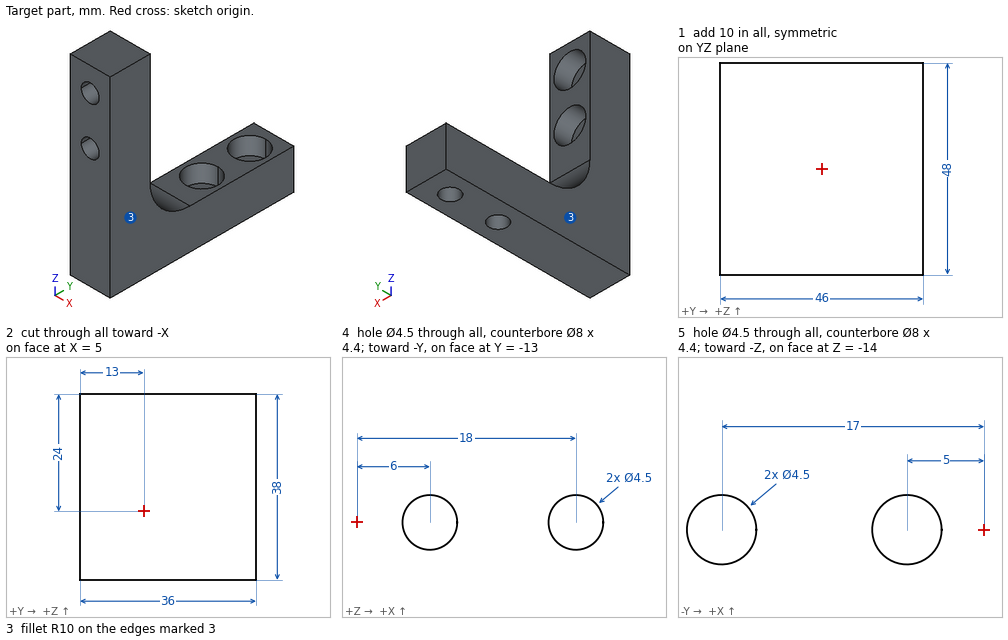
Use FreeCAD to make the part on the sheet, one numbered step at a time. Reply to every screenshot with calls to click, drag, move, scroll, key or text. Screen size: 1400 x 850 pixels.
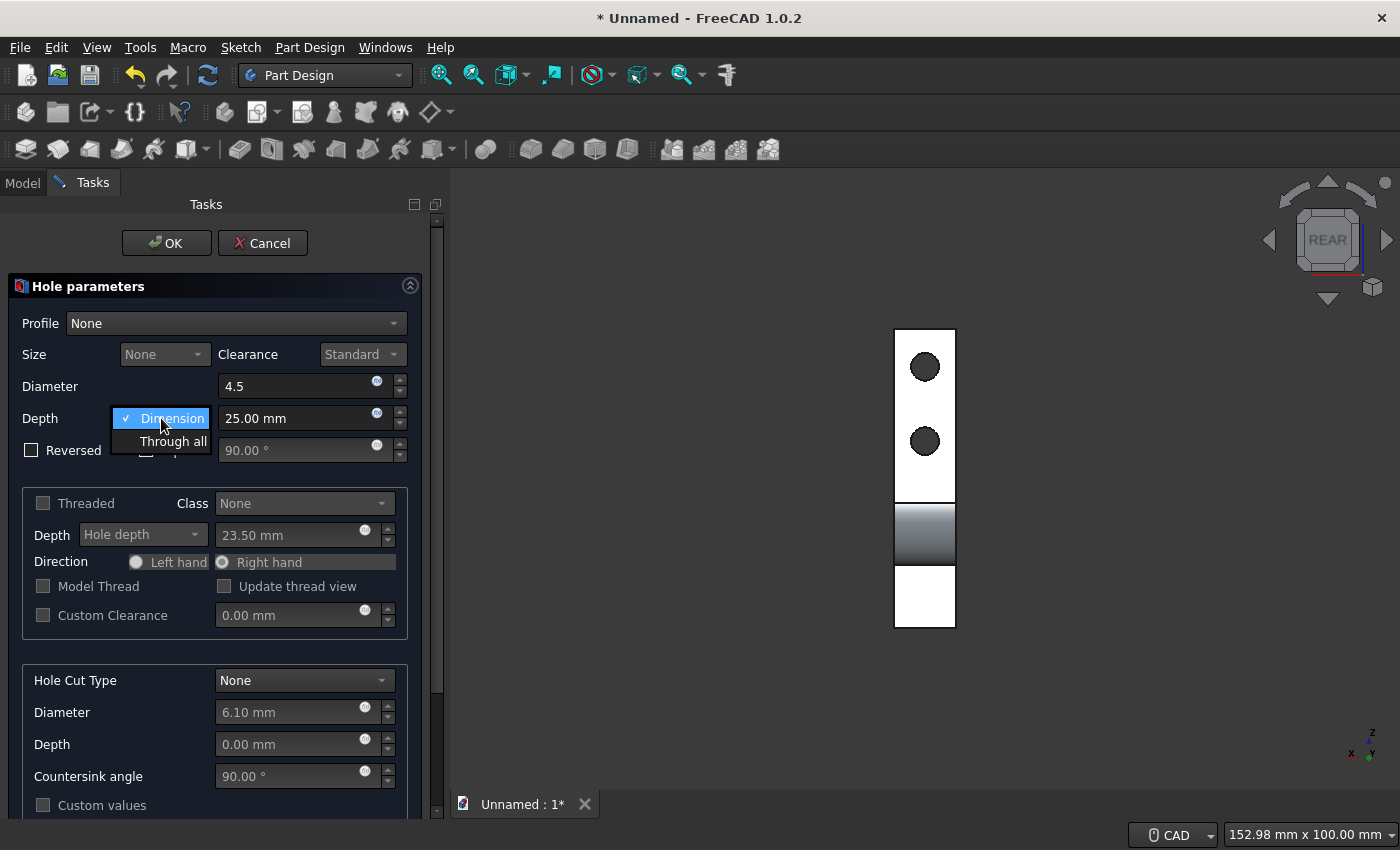
click(160, 442)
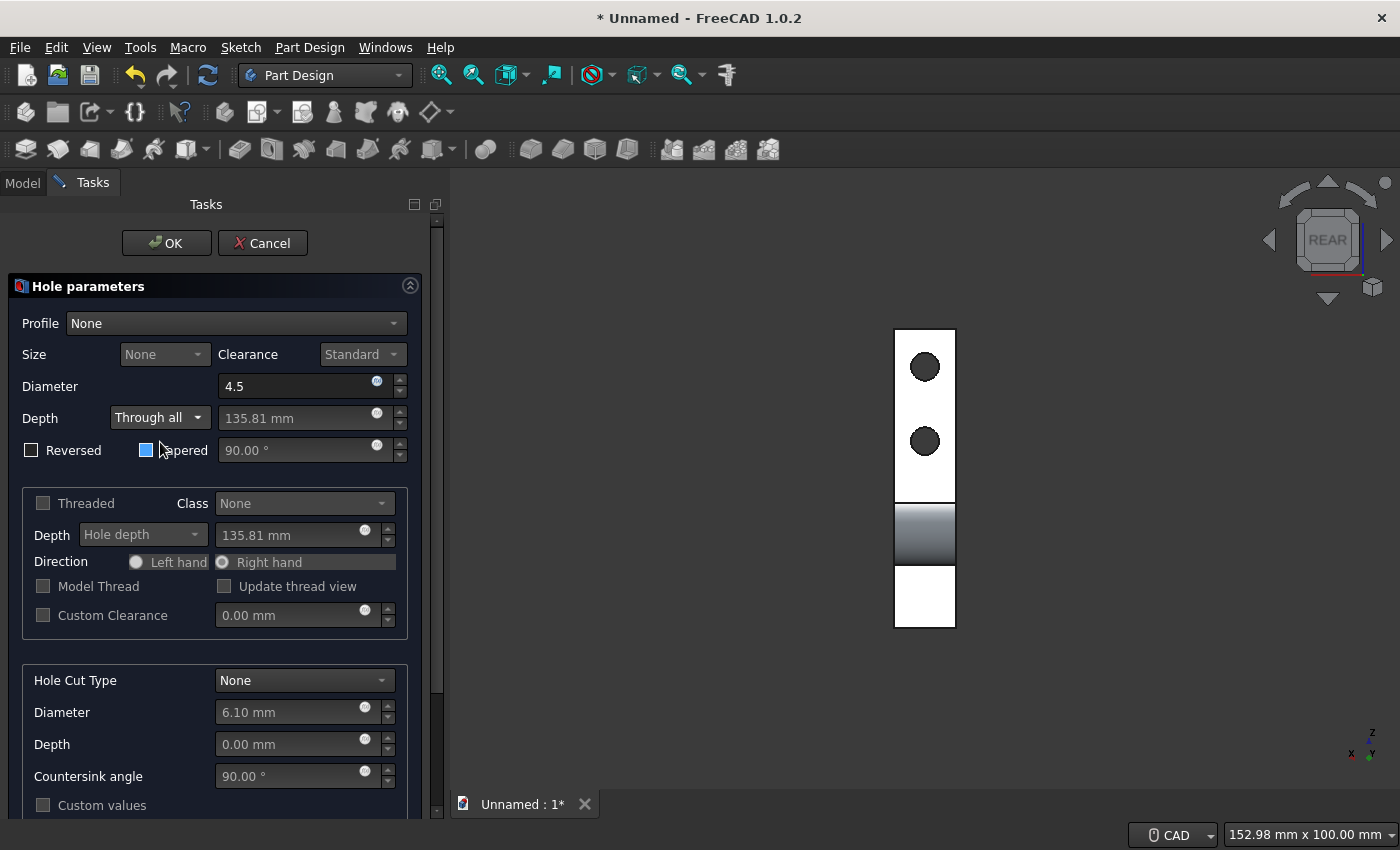
click(306, 680)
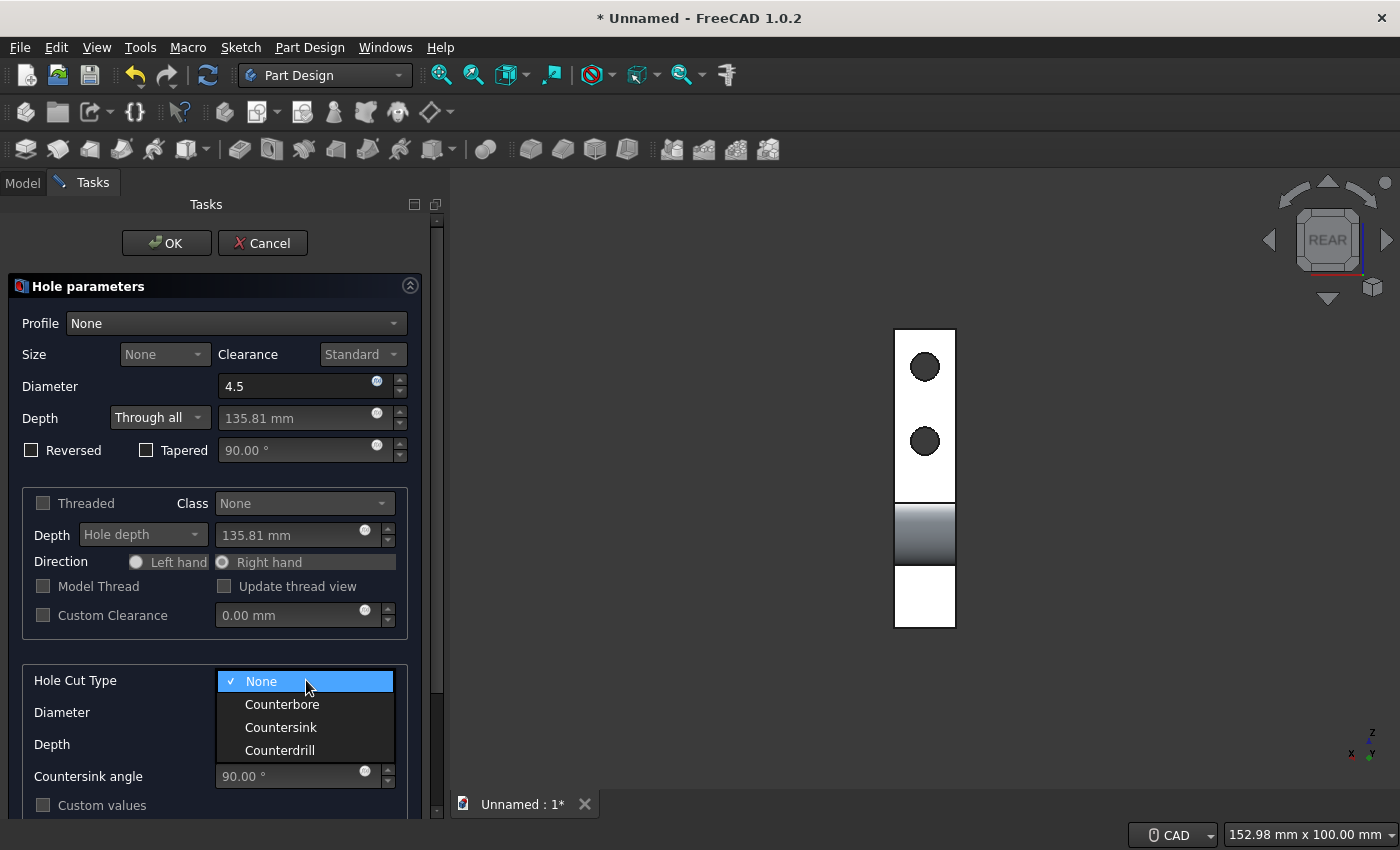
click(304, 704)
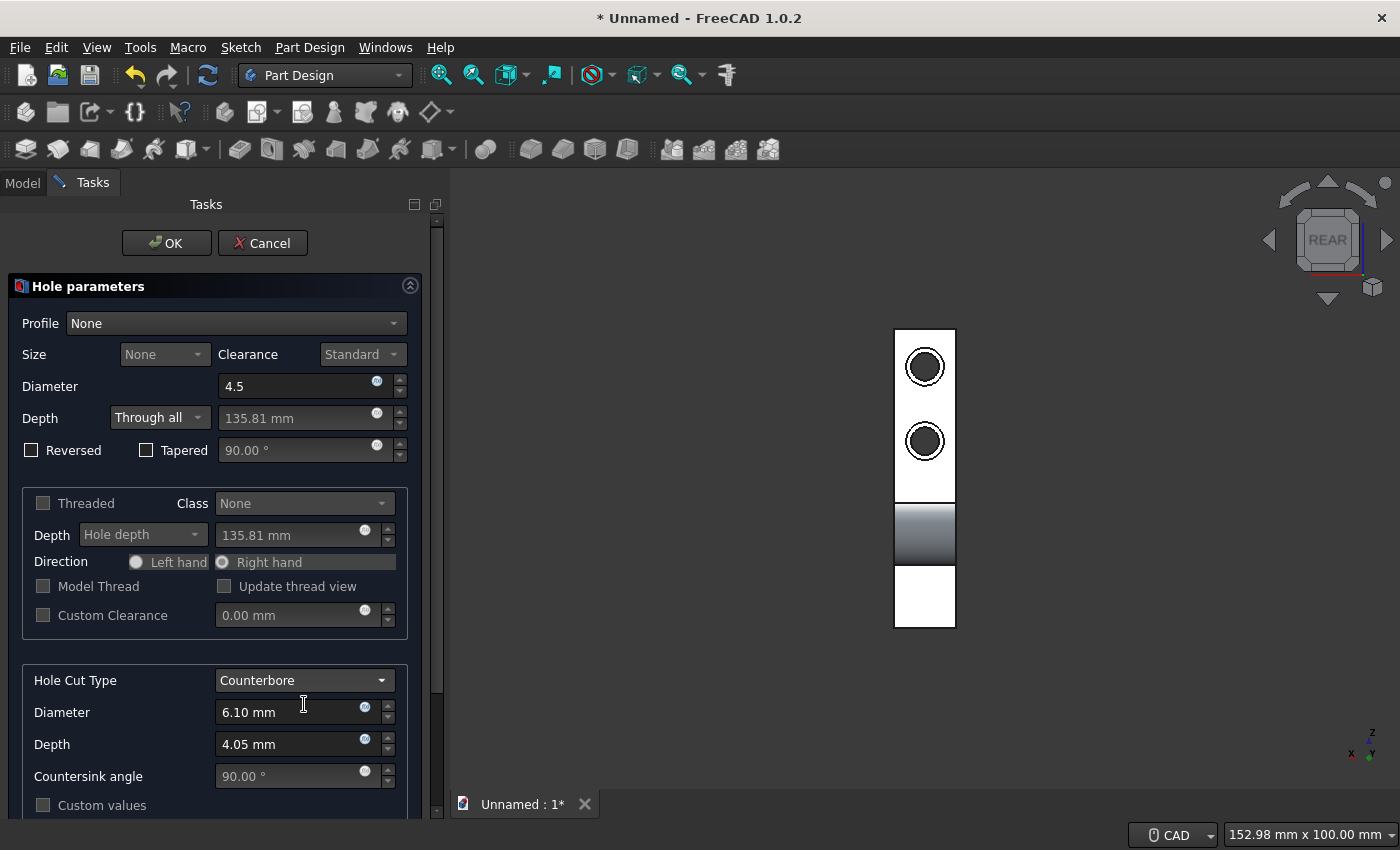
triple_click(298, 712)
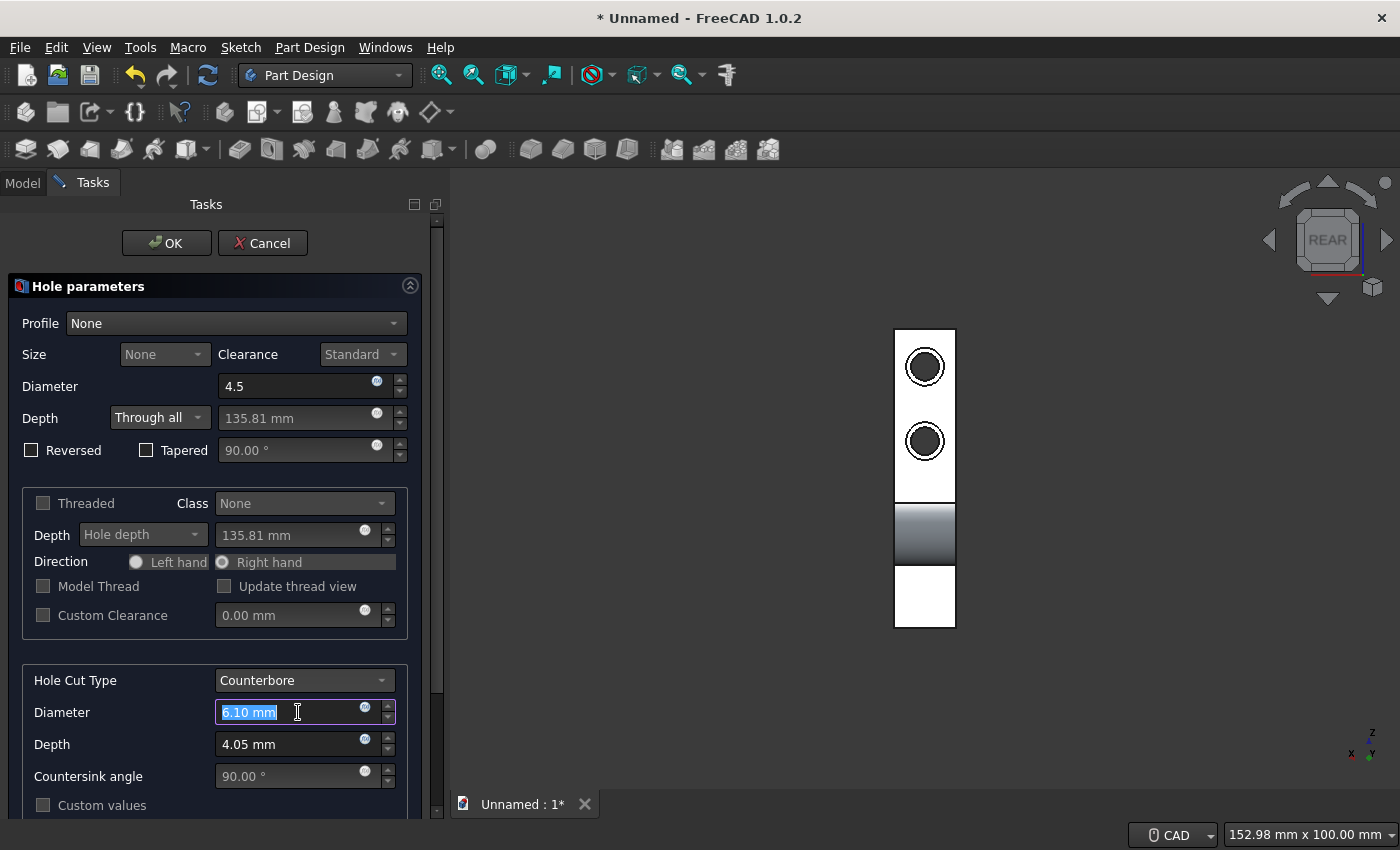
text(8)
key(Tab)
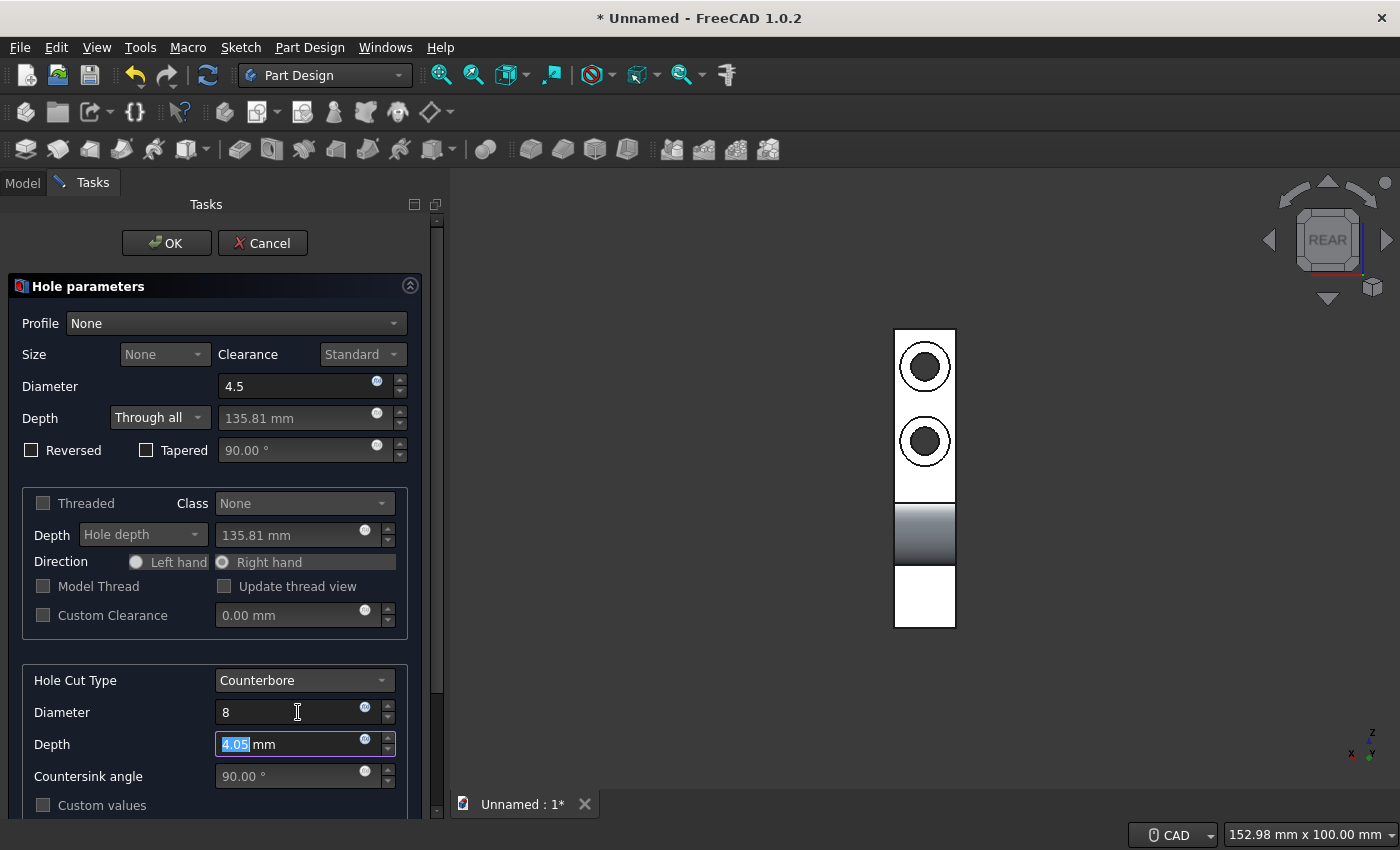
text(4.4)
key(Tab)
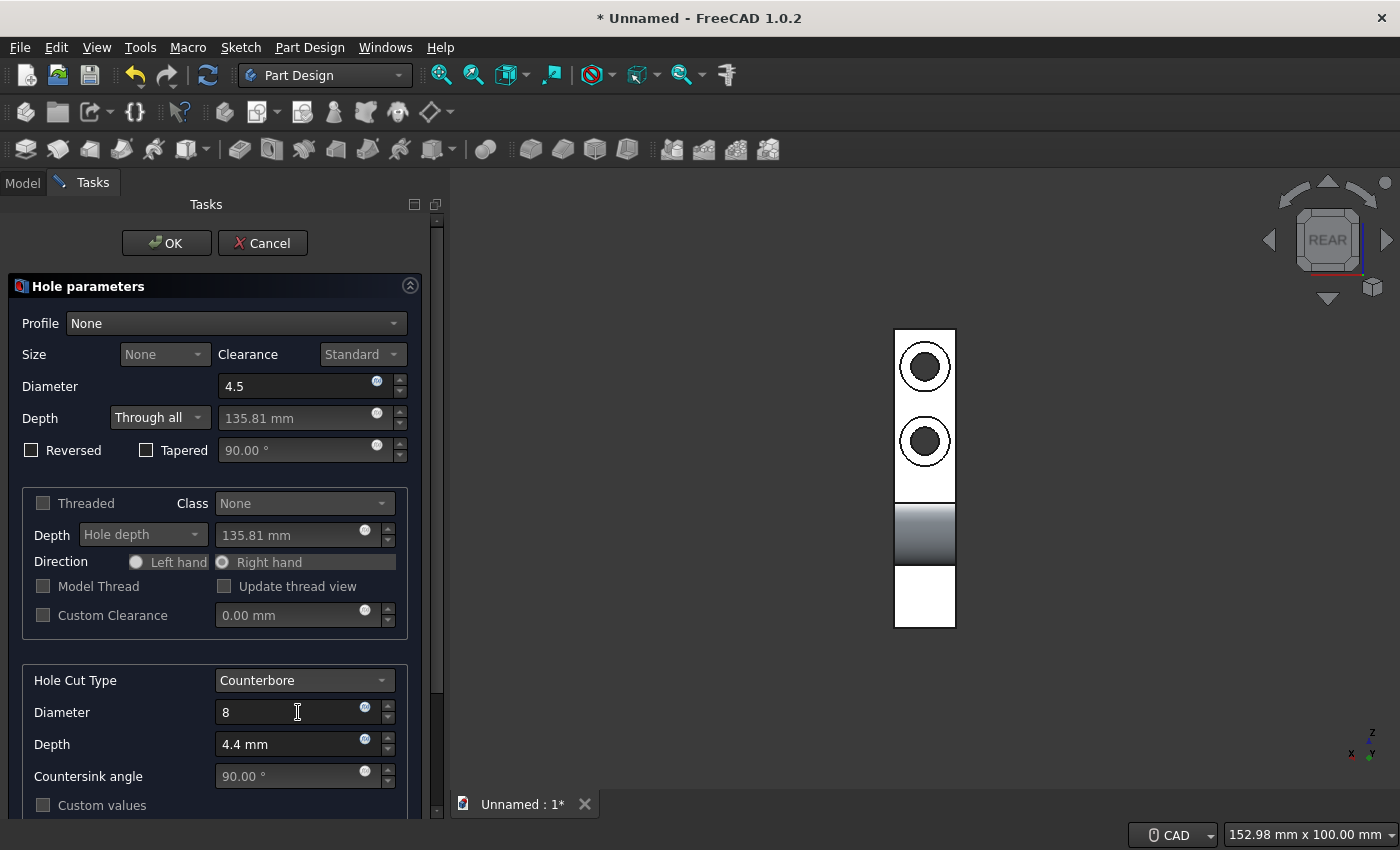
click(167, 243)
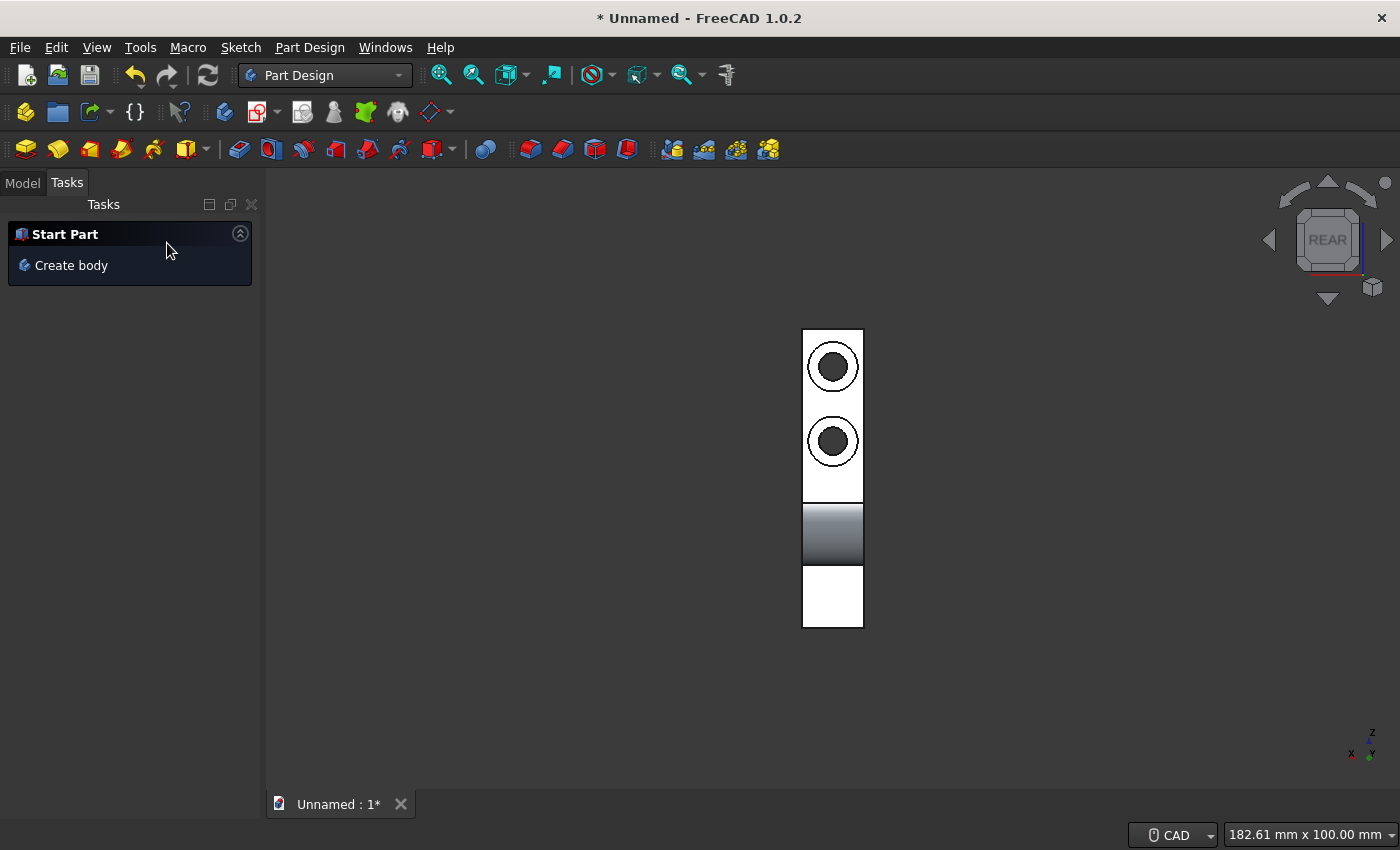
key(0)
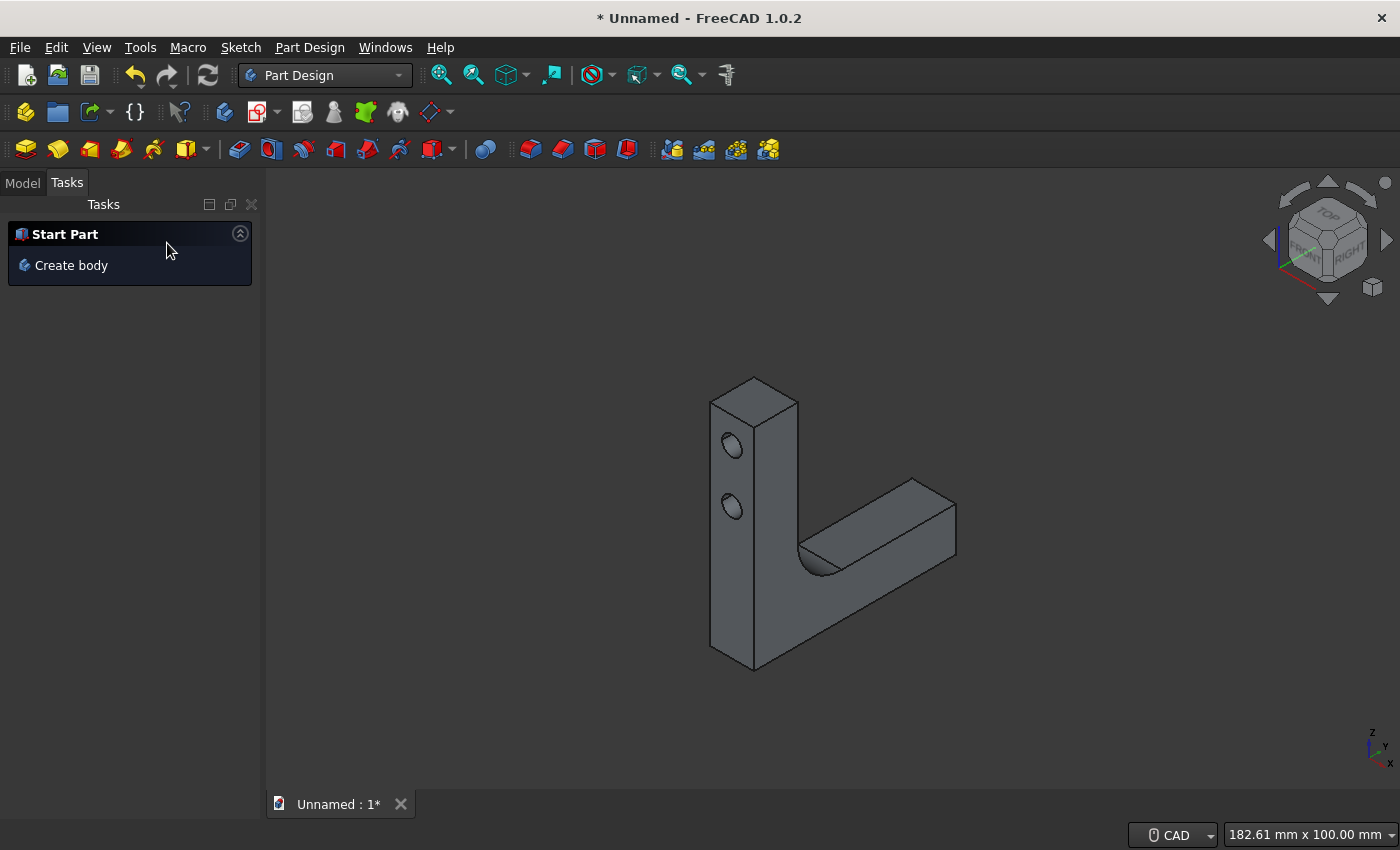
click(861, 533)